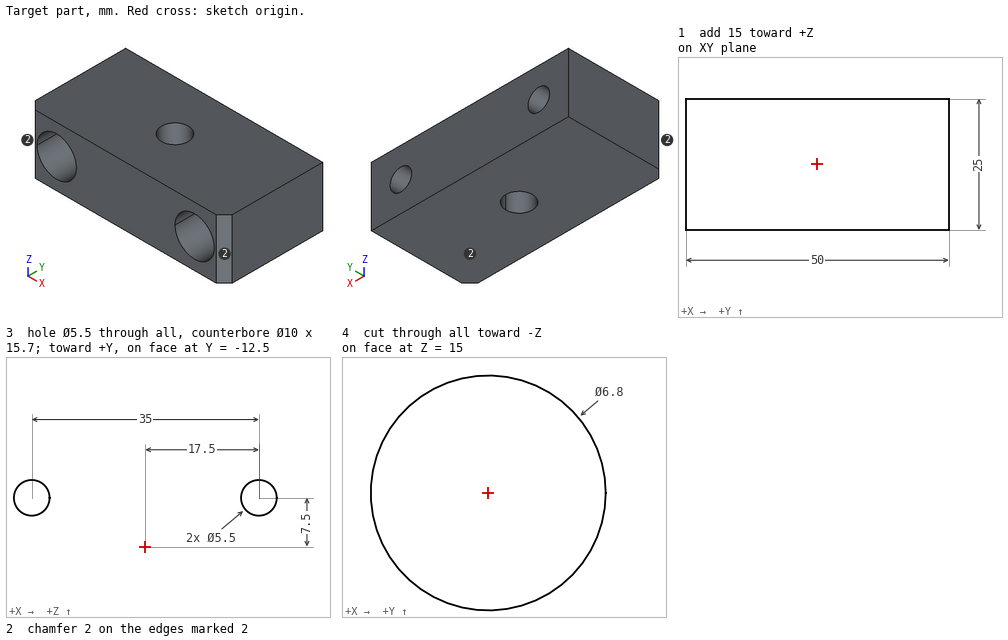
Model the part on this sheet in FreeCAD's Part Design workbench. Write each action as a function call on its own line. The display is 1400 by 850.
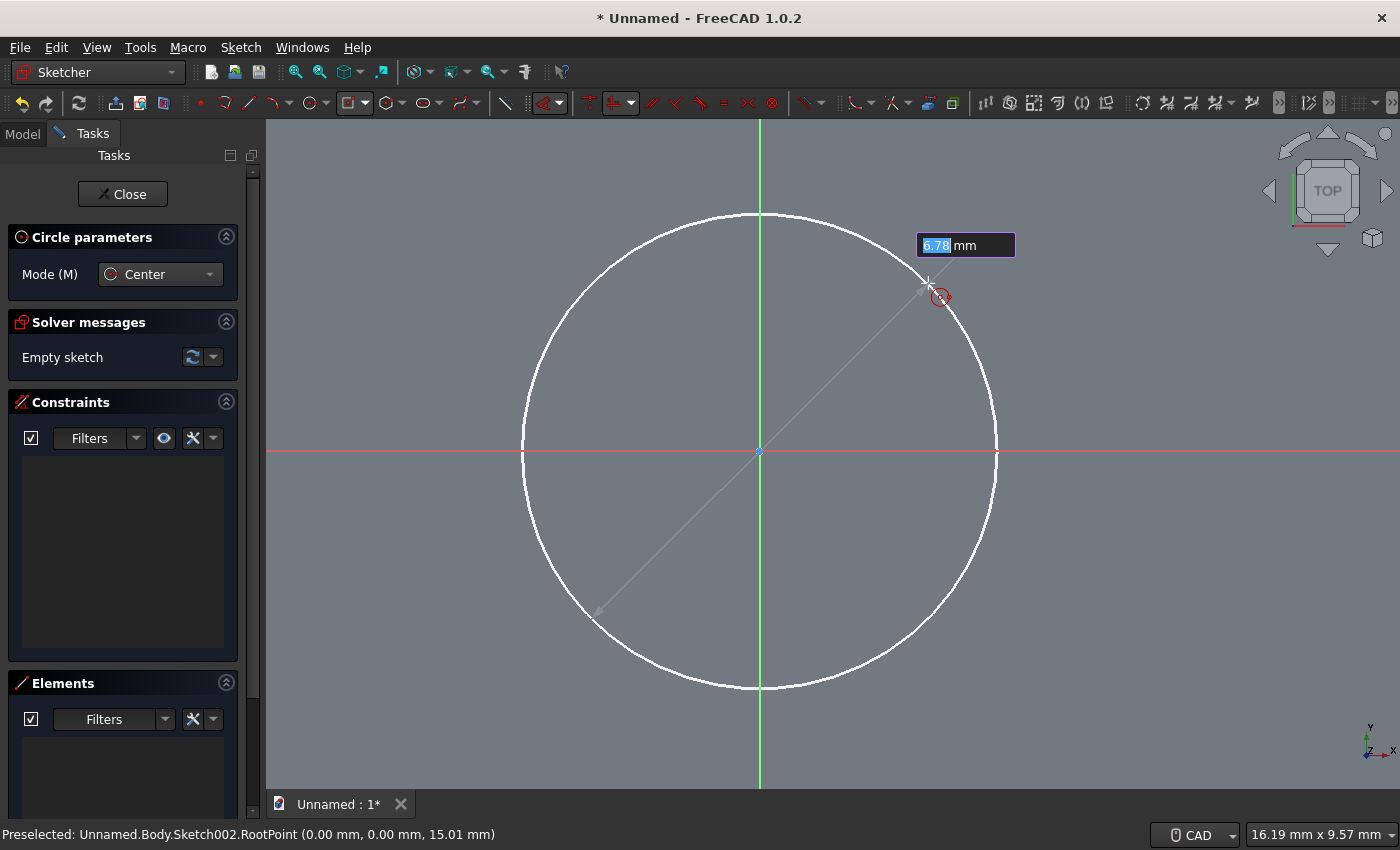
text(6.8)
key(Return)
key(Escape)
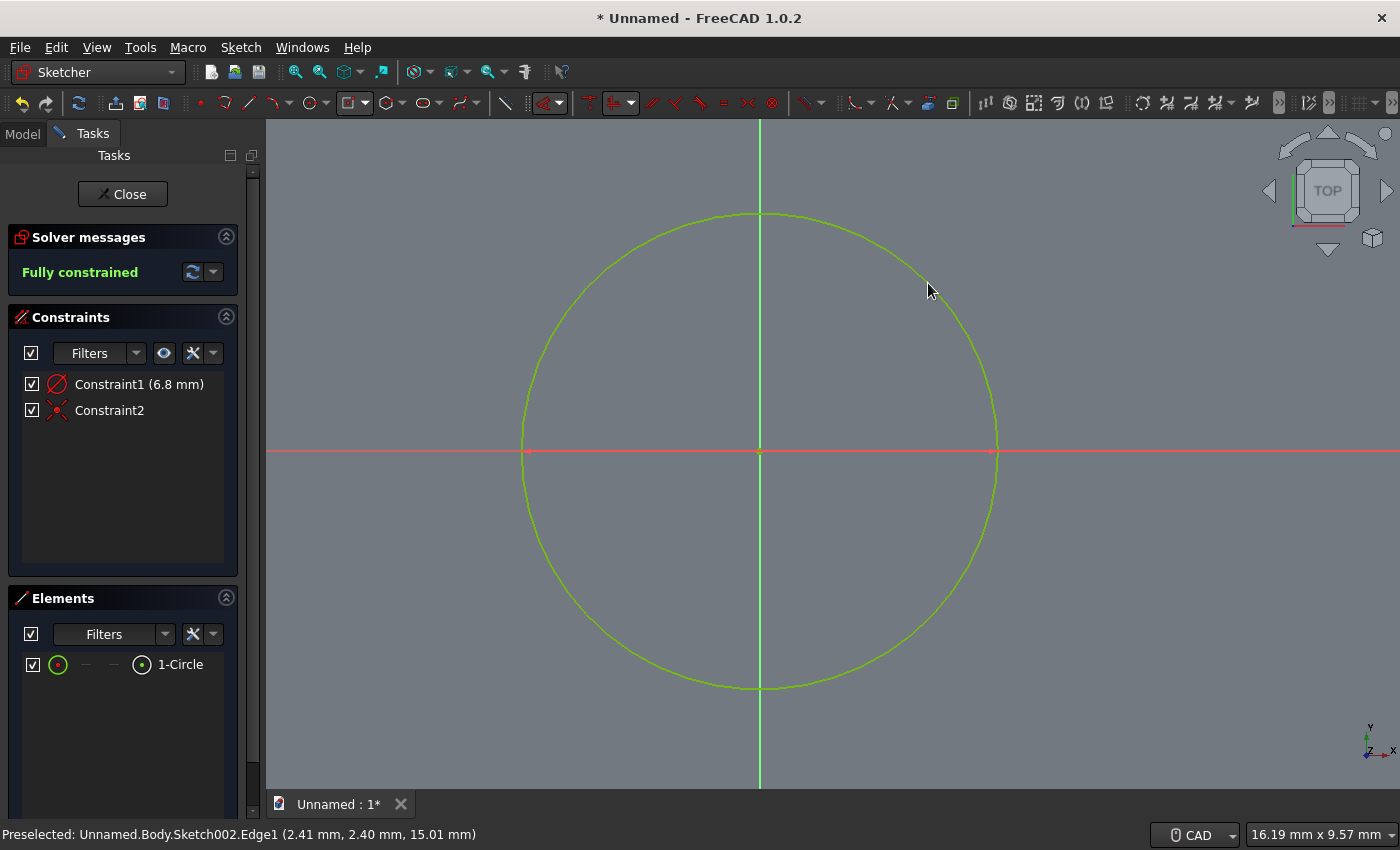
click(123, 194)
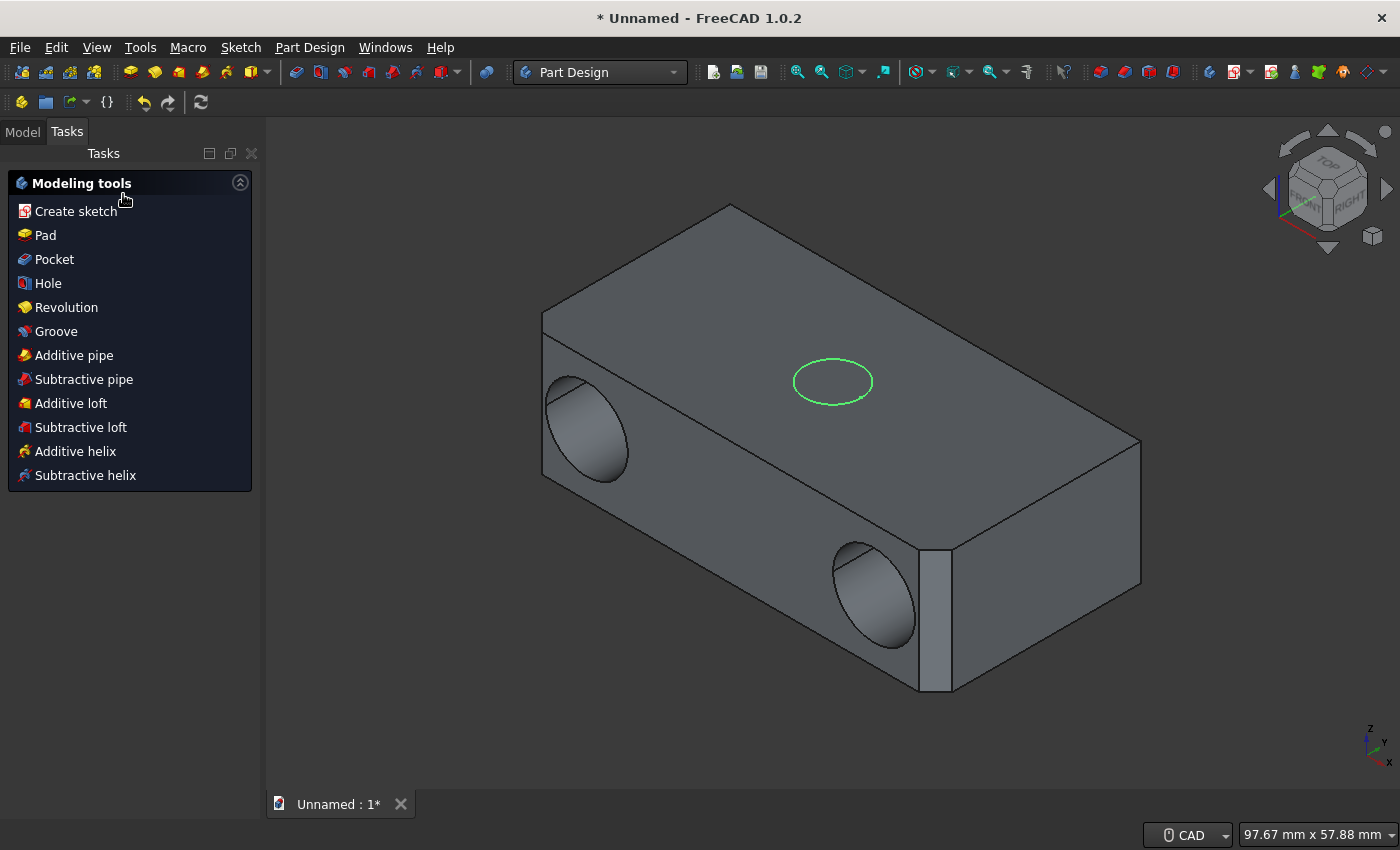
click(298, 72)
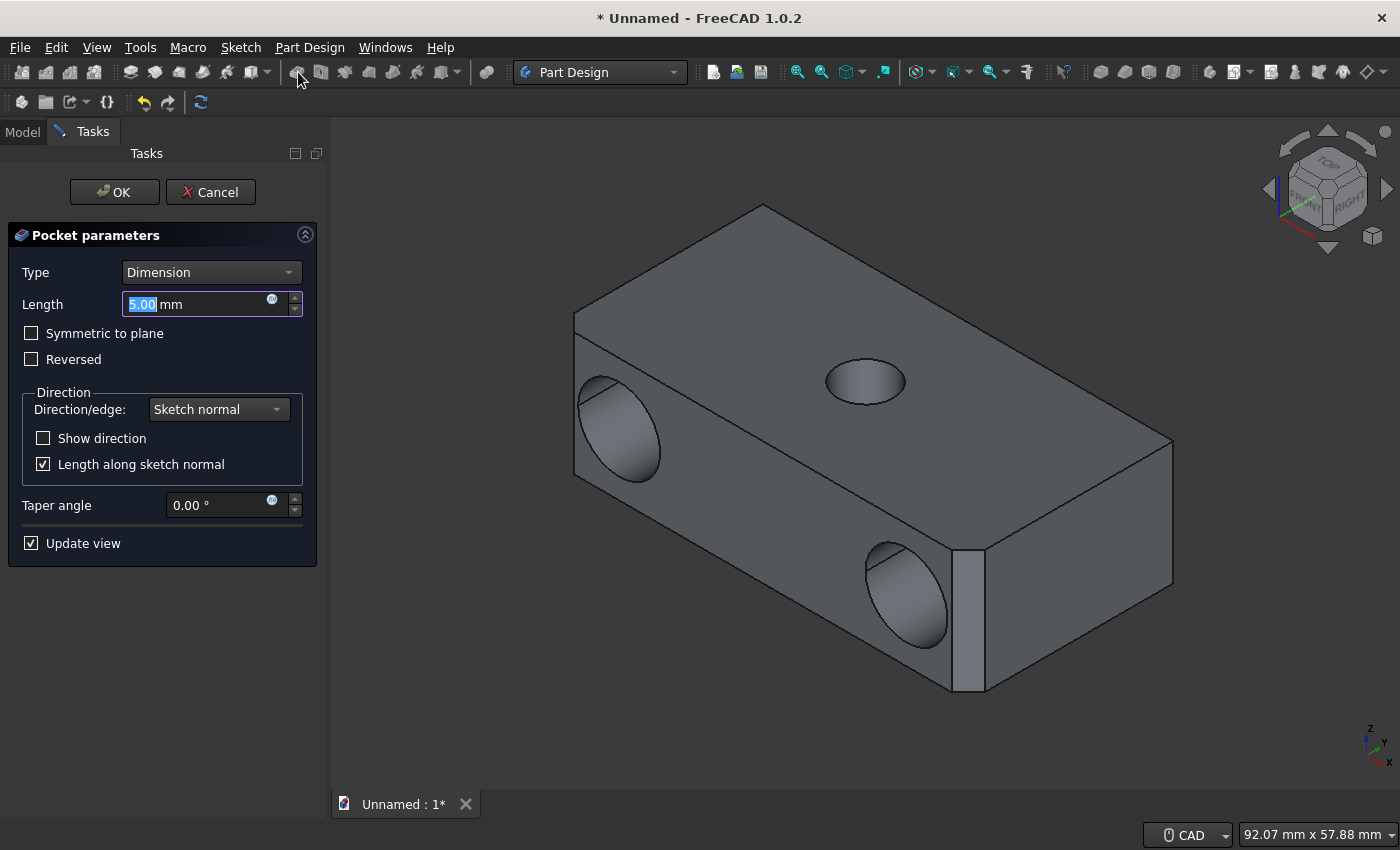
click(212, 272)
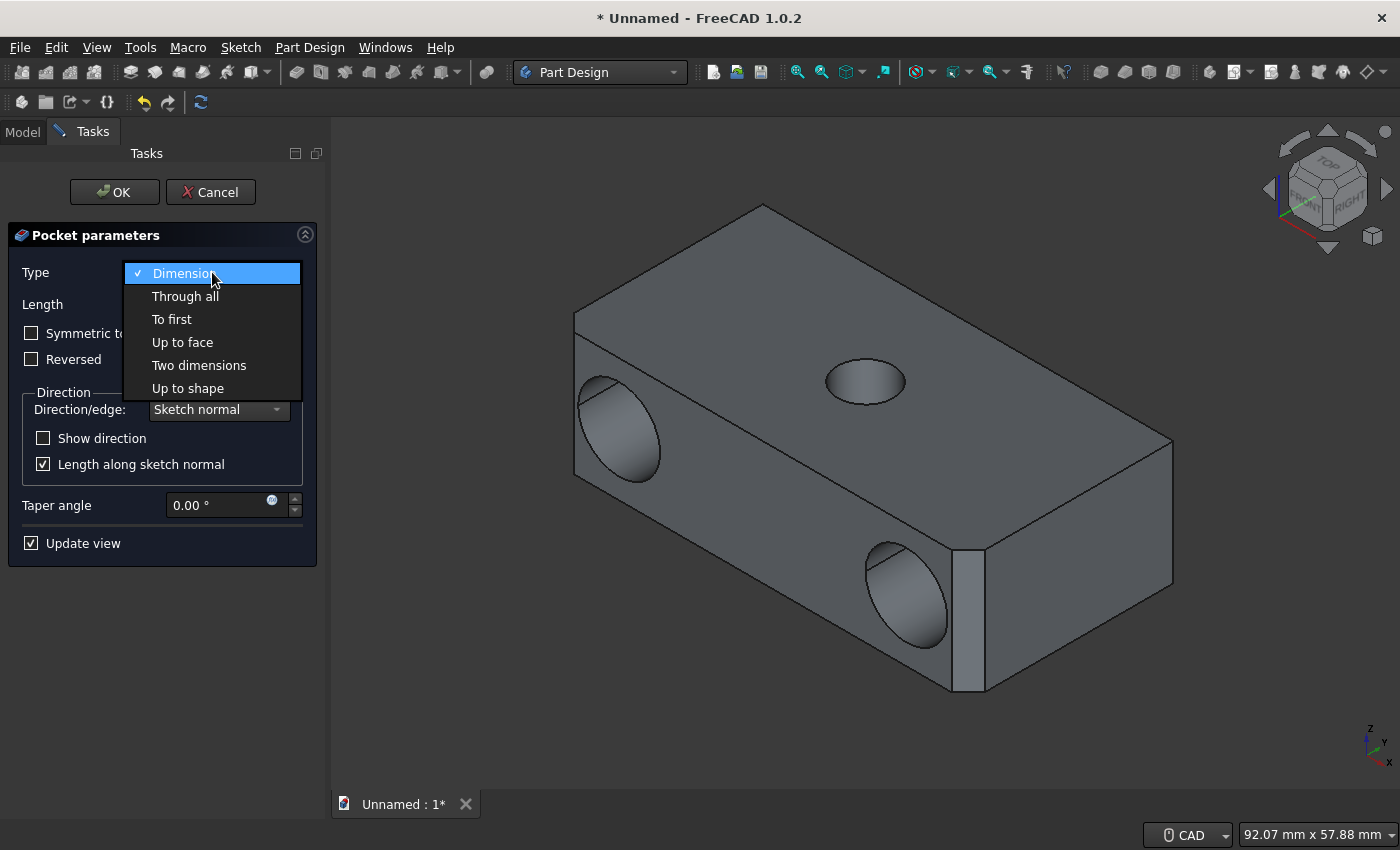
click(212, 296)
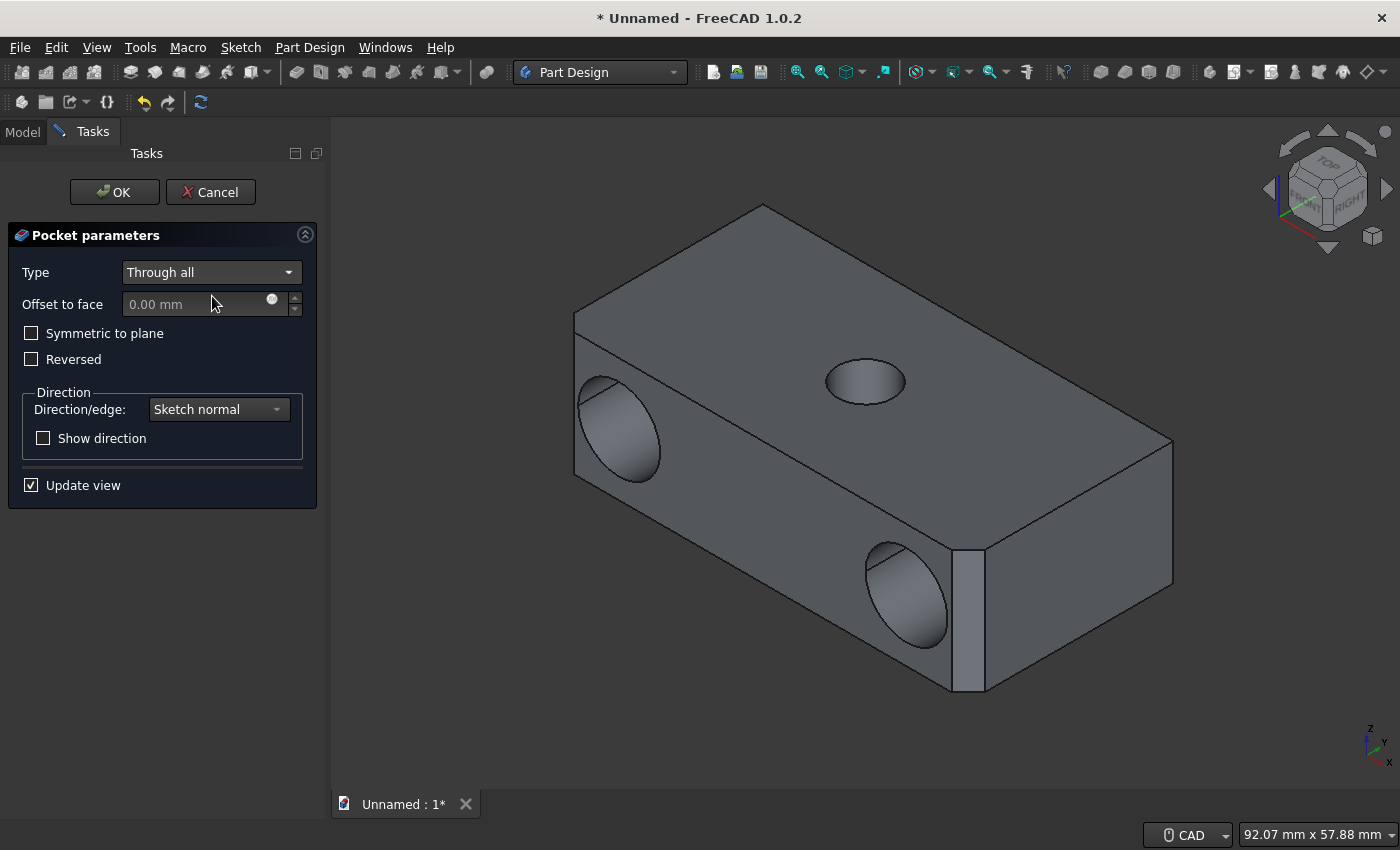
click(115, 192)